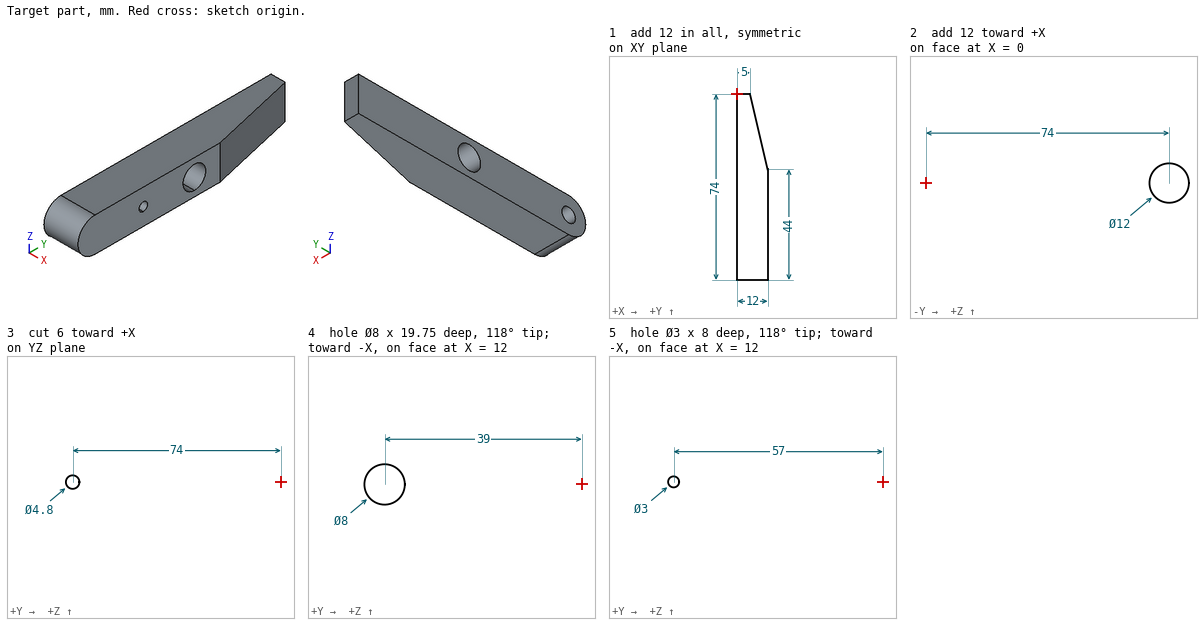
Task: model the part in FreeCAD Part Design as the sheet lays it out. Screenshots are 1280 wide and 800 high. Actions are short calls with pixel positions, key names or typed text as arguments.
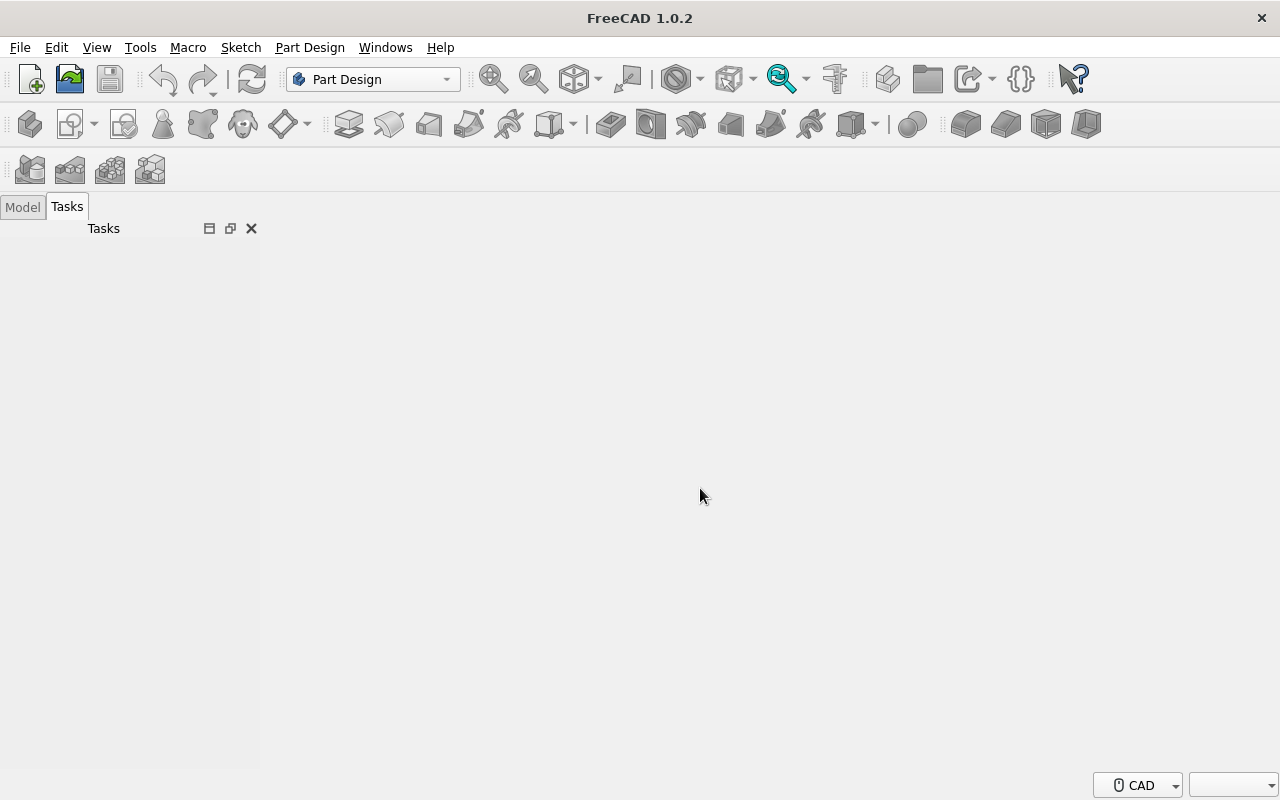
click(30, 80)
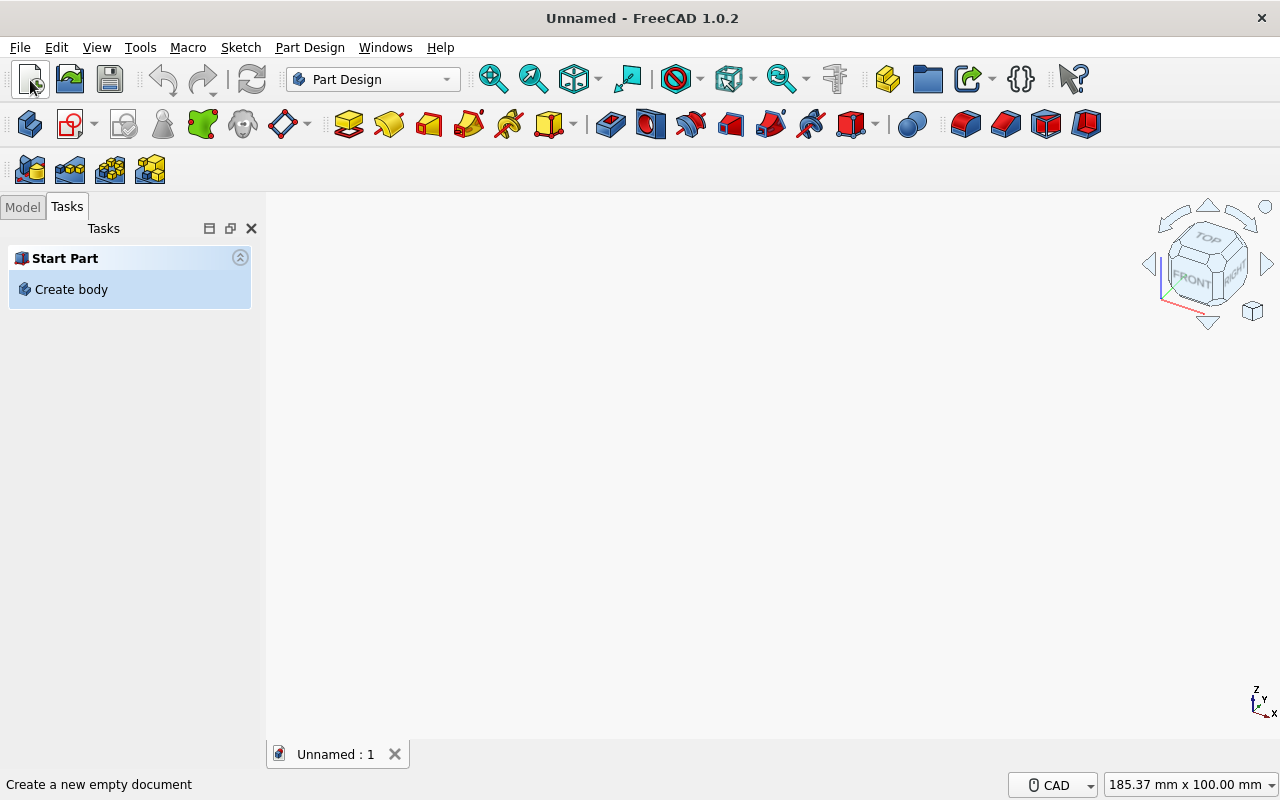
click(70, 124)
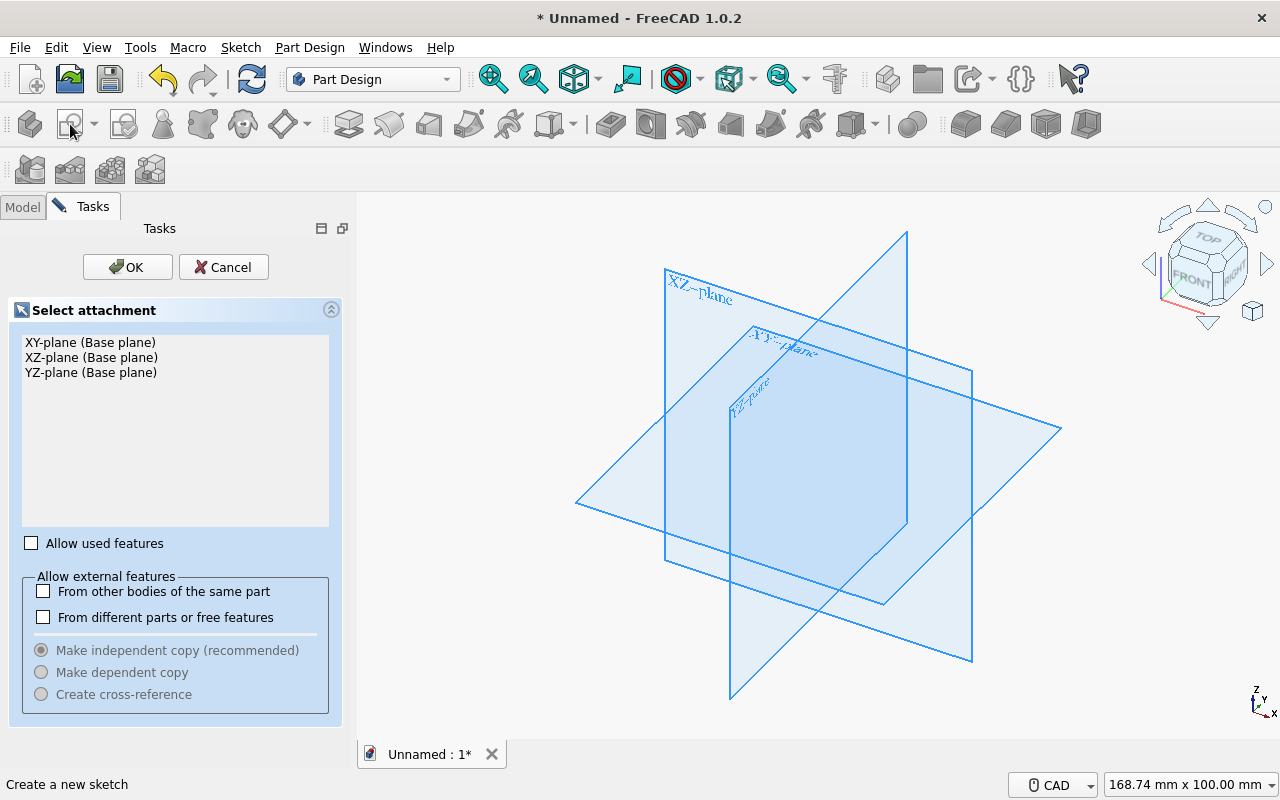
click(82, 342)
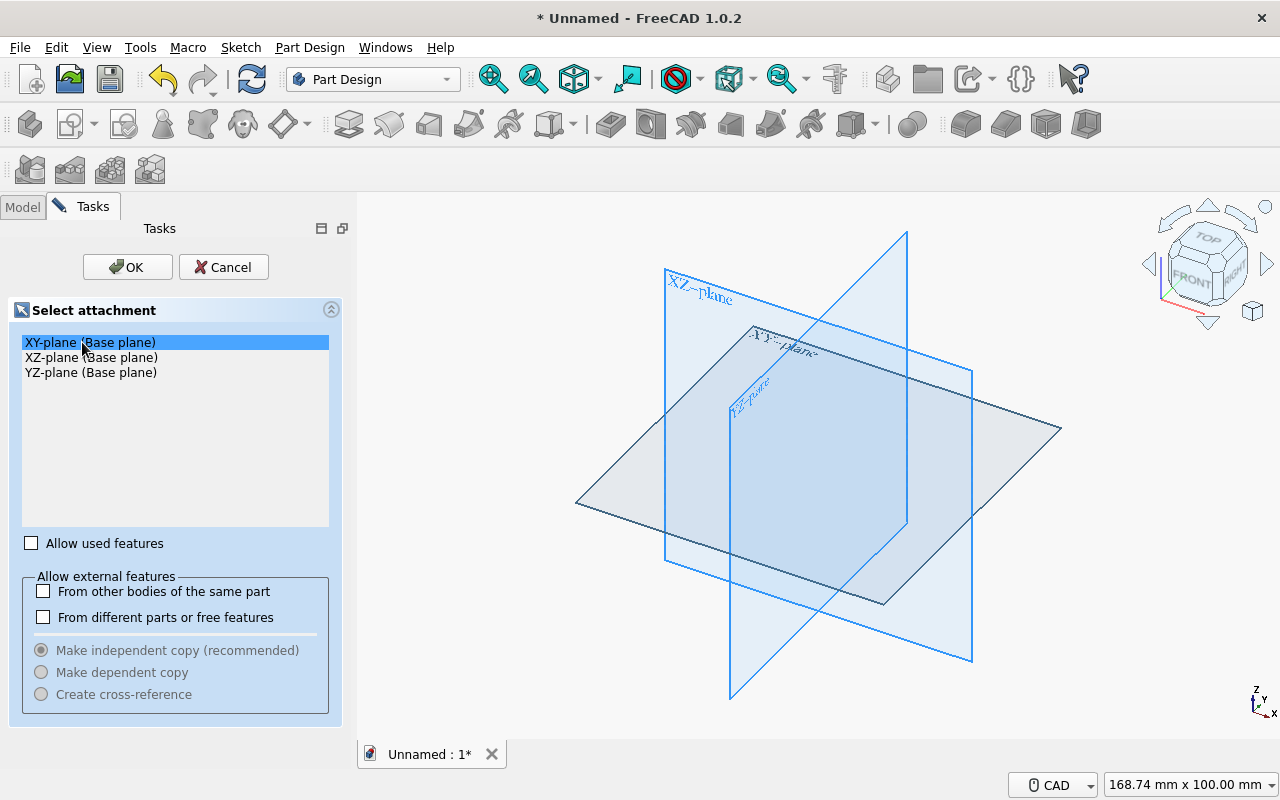
click(128, 267)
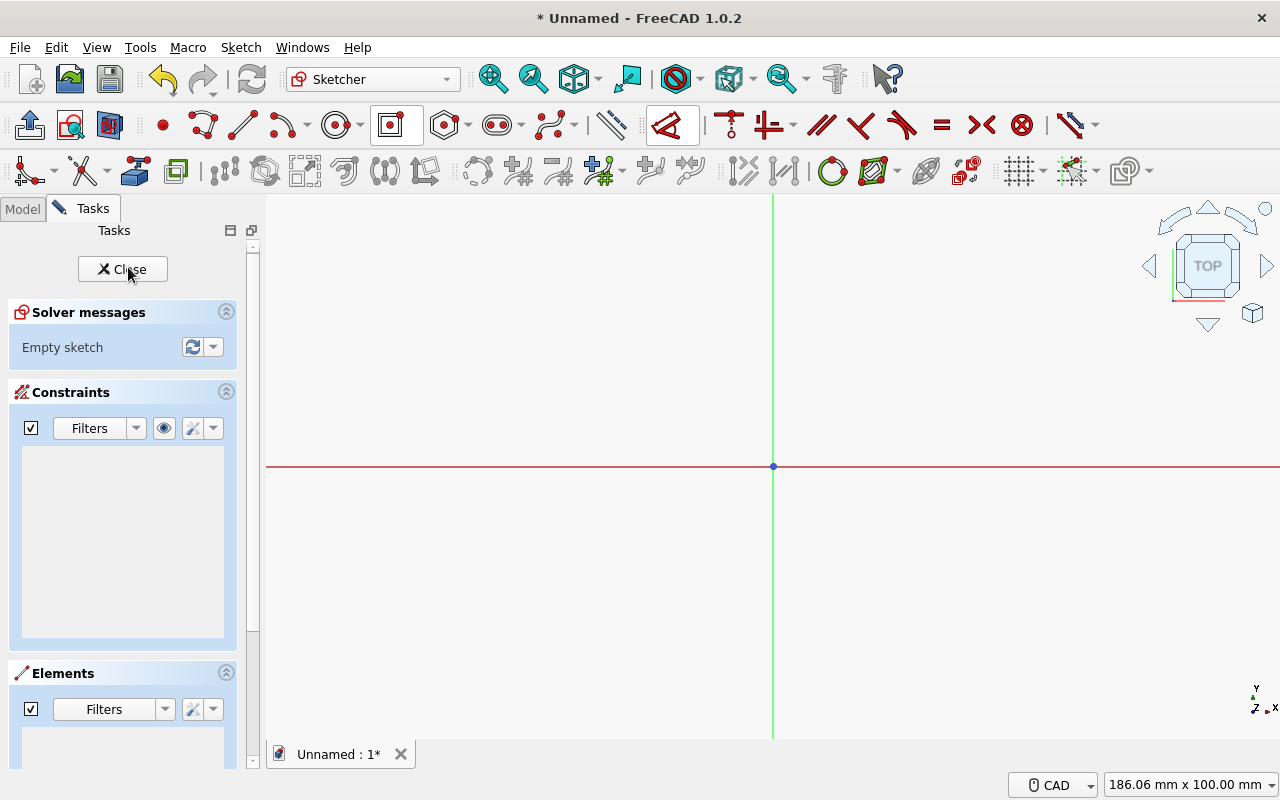
scroll(499, 222, down, 2)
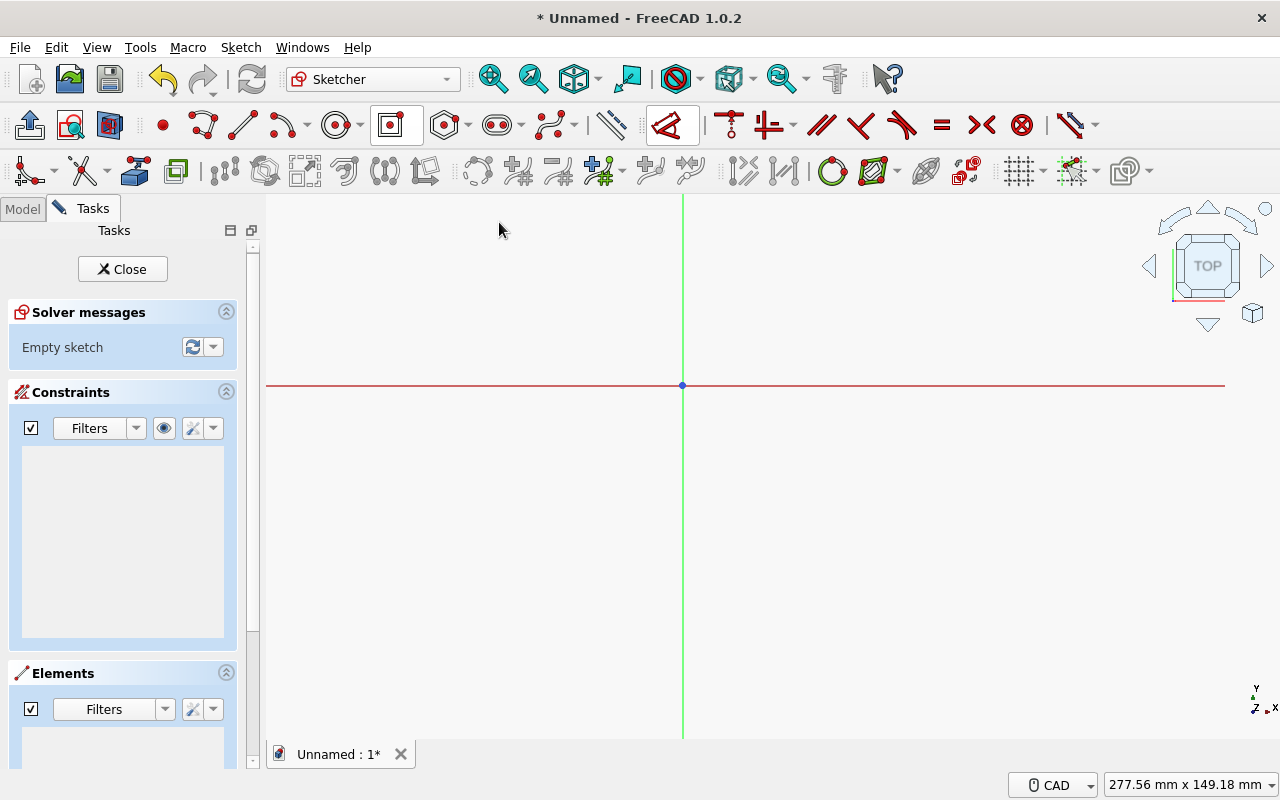
click(204, 126)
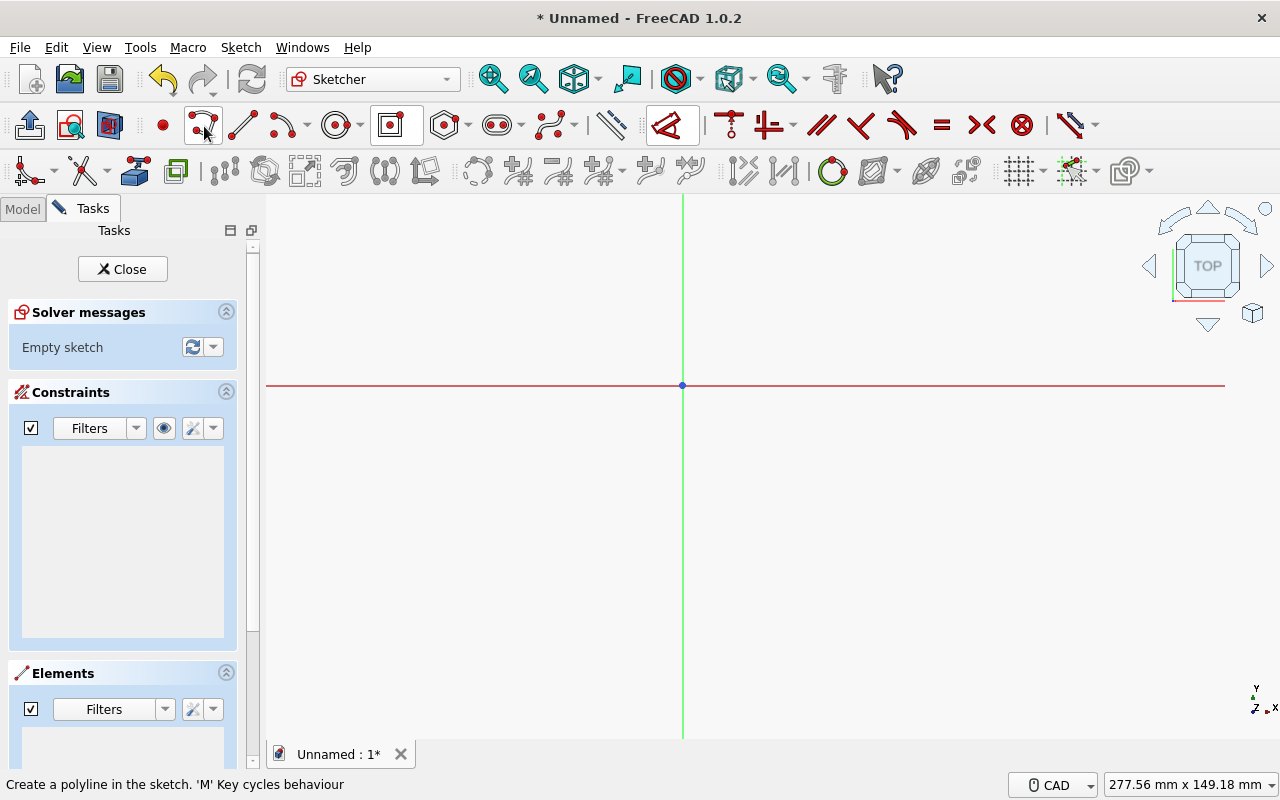
click(683, 386)
click(692, 656)
click(727, 656)
click(727, 496)
click(701, 395)
click(683, 386)
key(Escape)
key(Escape)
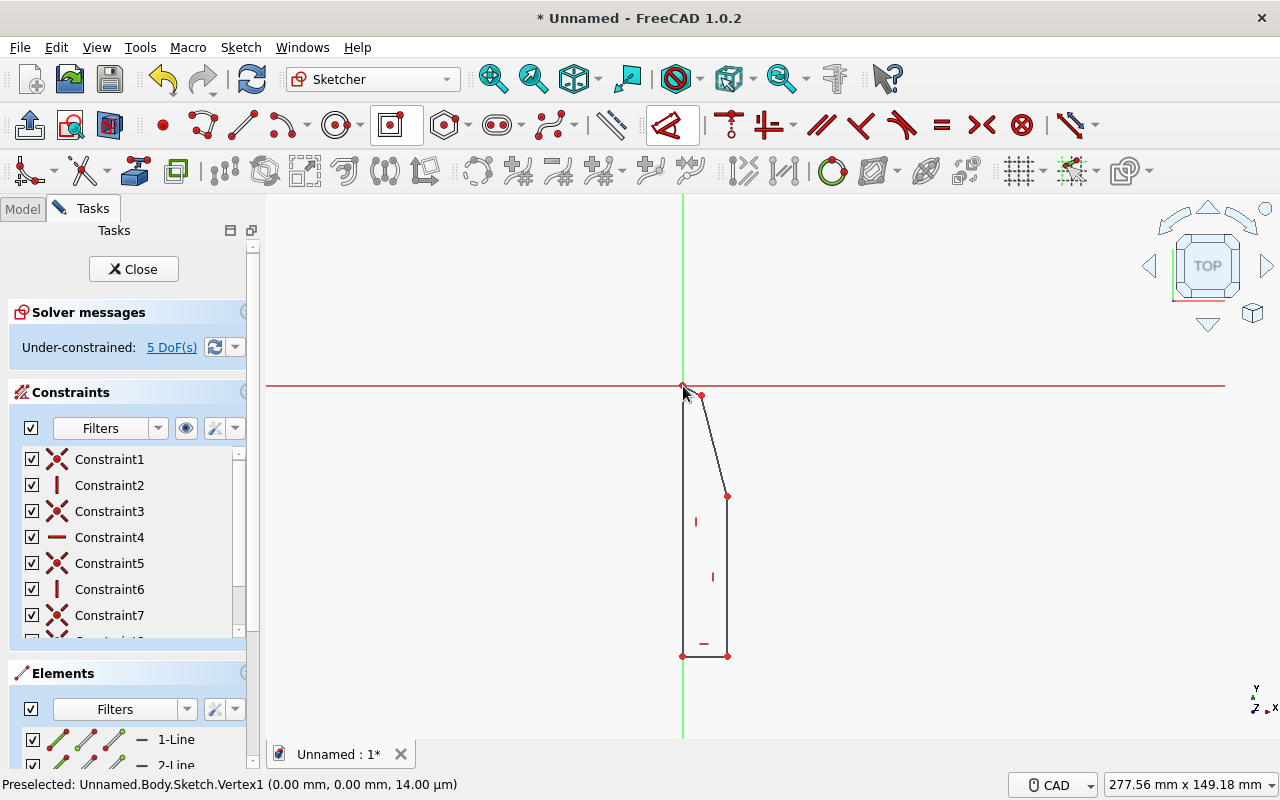
scroll(696, 393, up, 4)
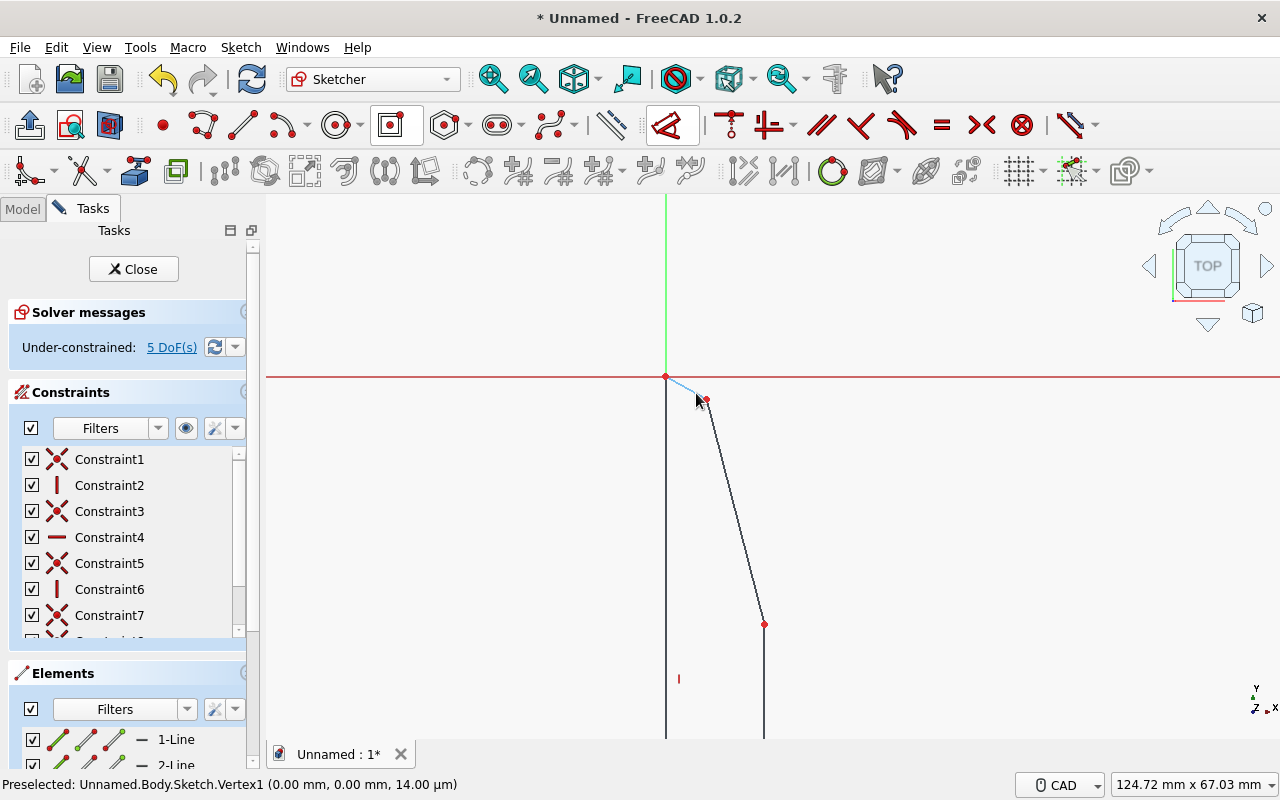
click(694, 392)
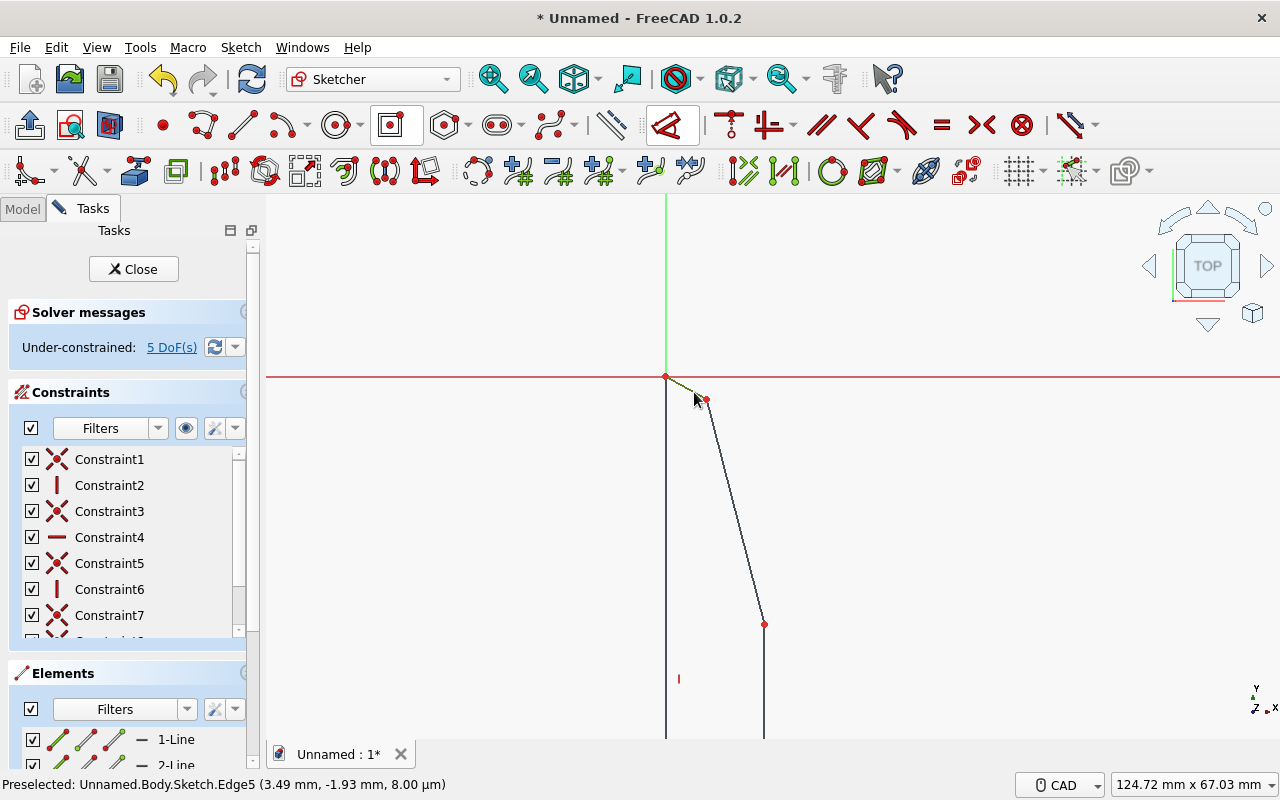
click(796, 126)